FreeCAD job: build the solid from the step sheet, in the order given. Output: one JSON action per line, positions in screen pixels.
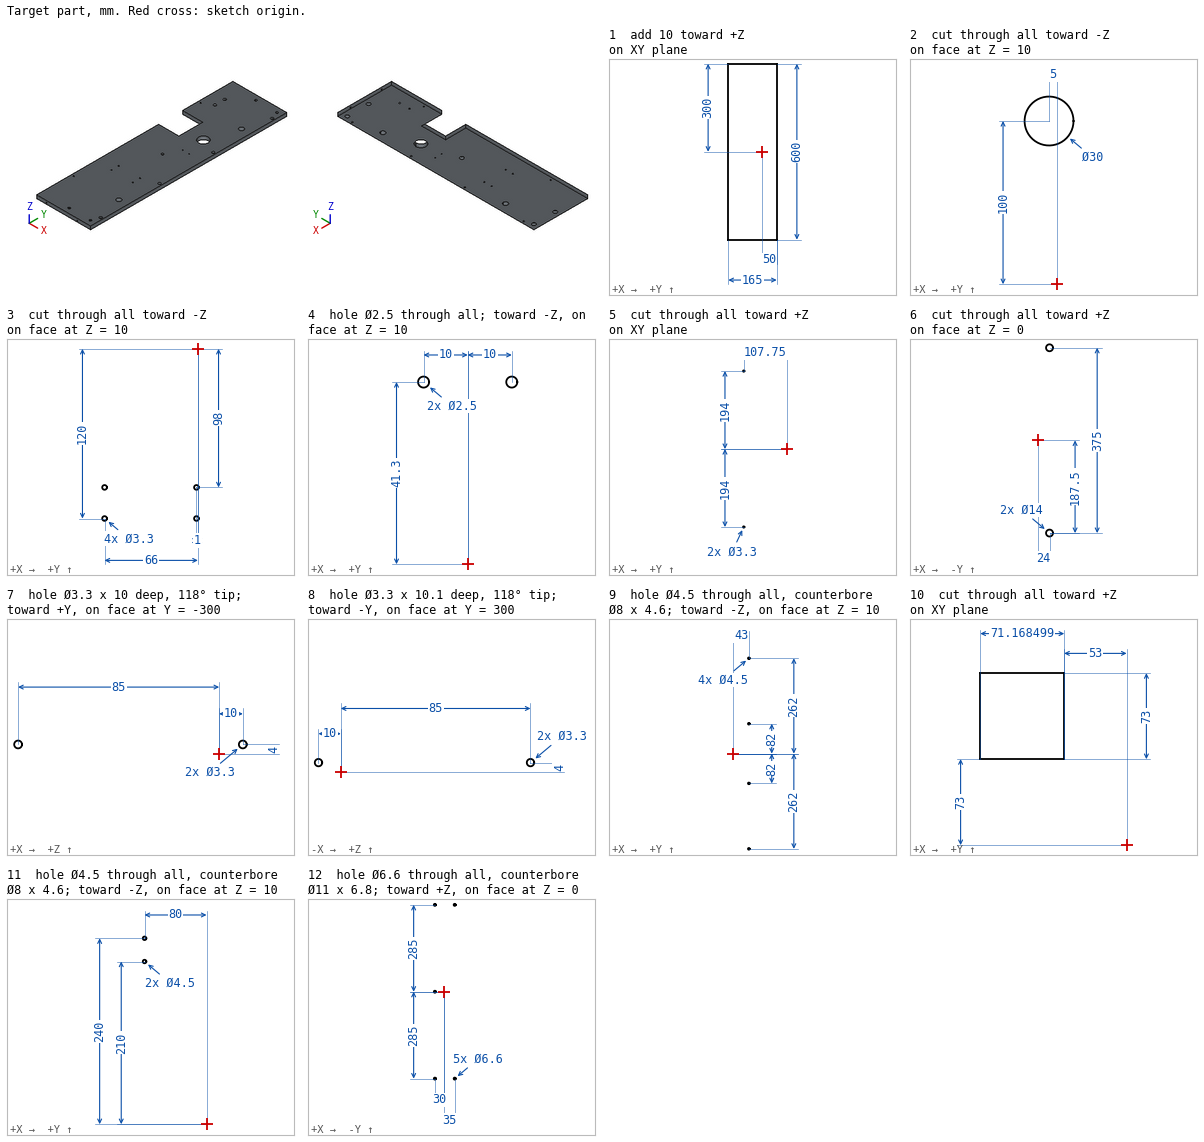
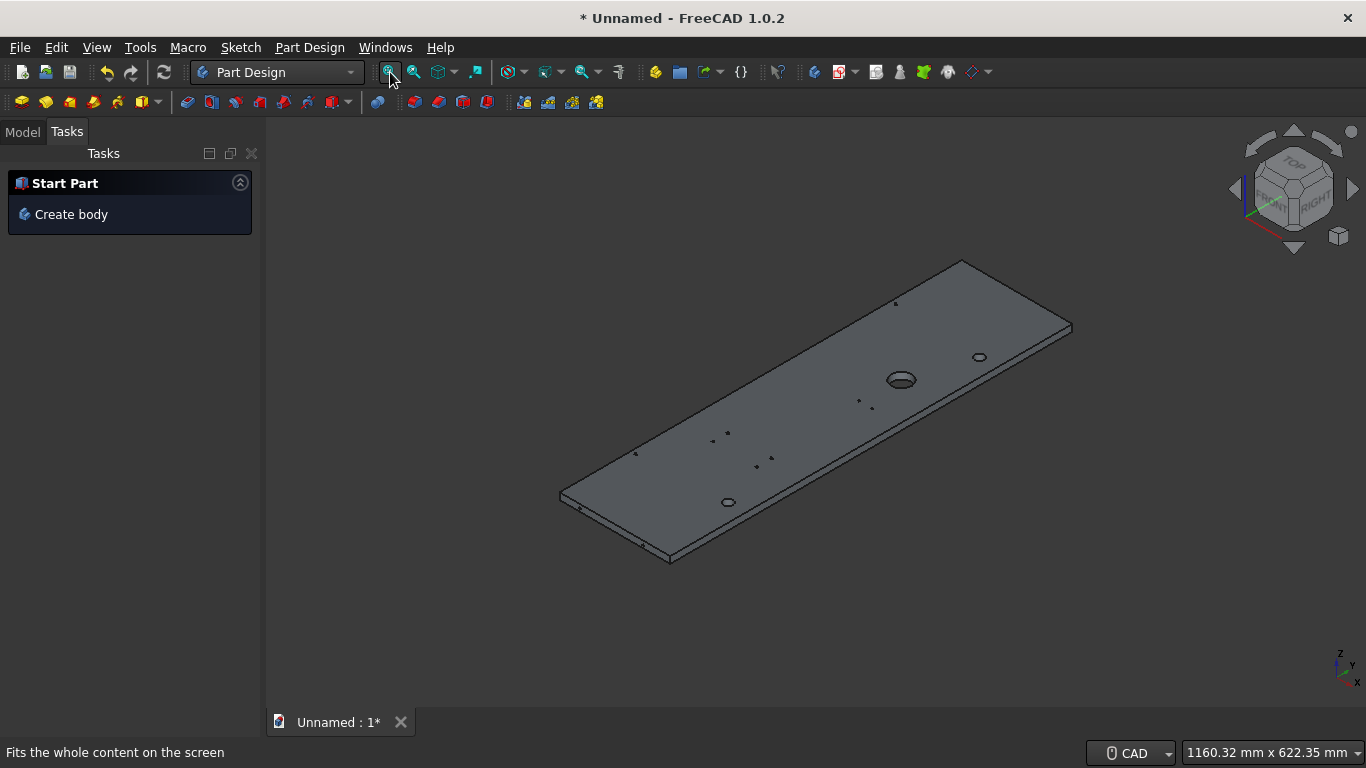
{"action": "left_click", "coordinate": [800, 398]}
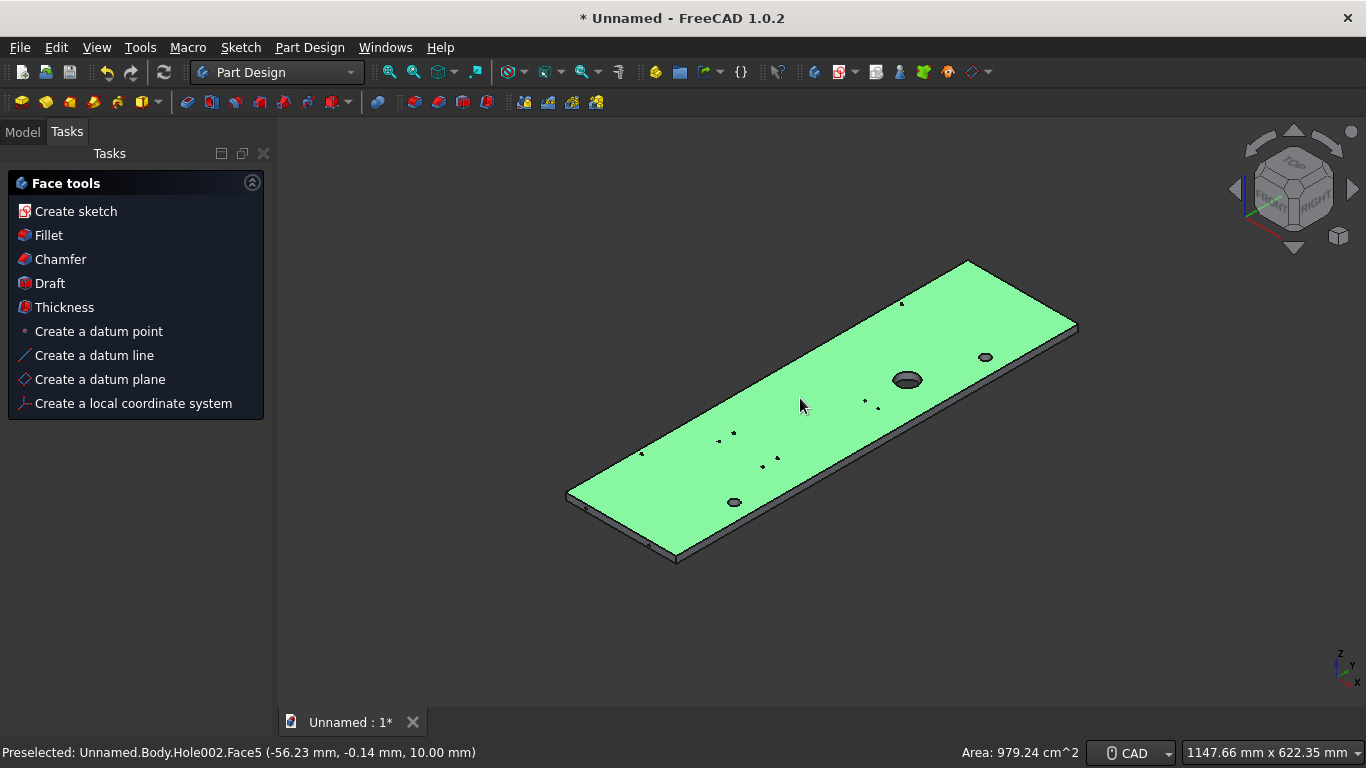
{"action": "left_click", "coordinate": [840, 72]}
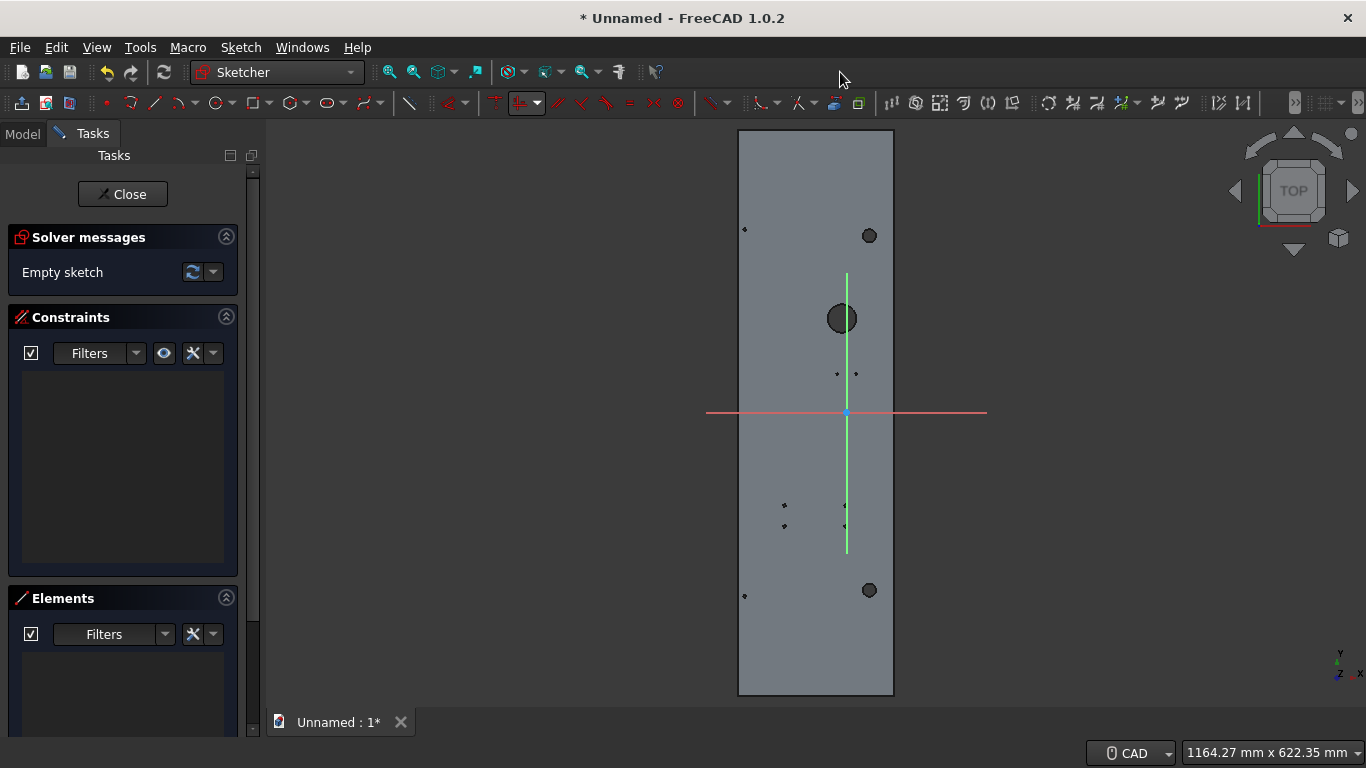
{"action": "scroll", "coordinate": [294, 413], "scroll_direction": "down", "scroll_amount": 1}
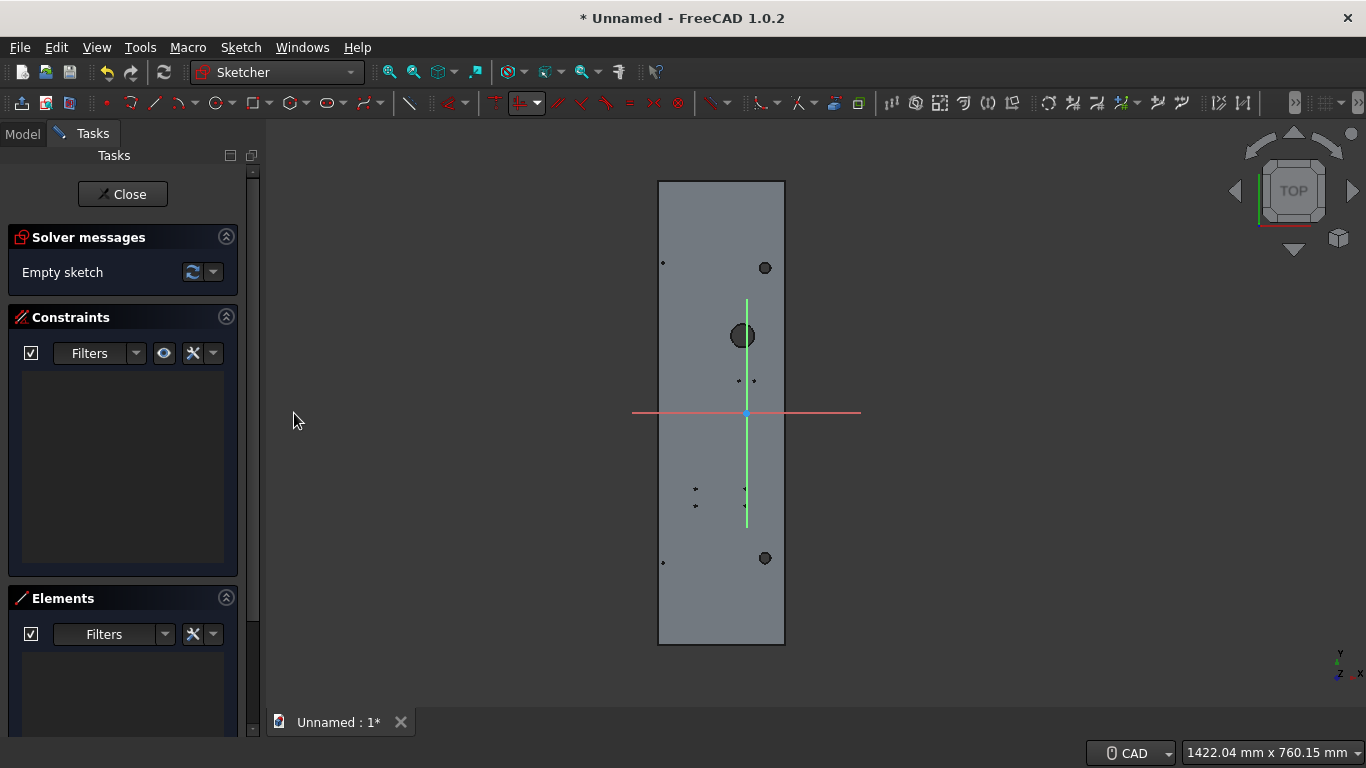
{"action": "left_click", "coordinate": [216, 104]}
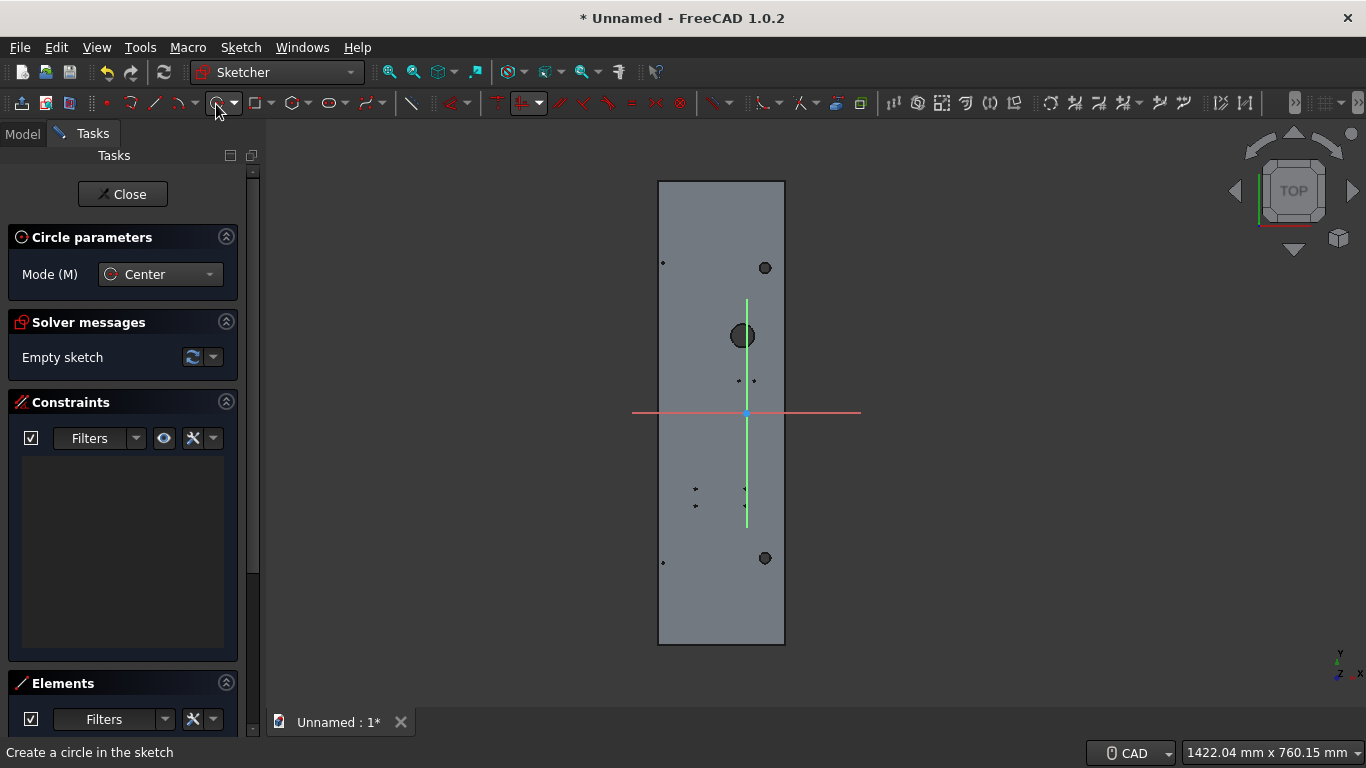
{"action": "scroll", "coordinate": [780, 210], "scroll_direction": "up", "scroll_amount": 13}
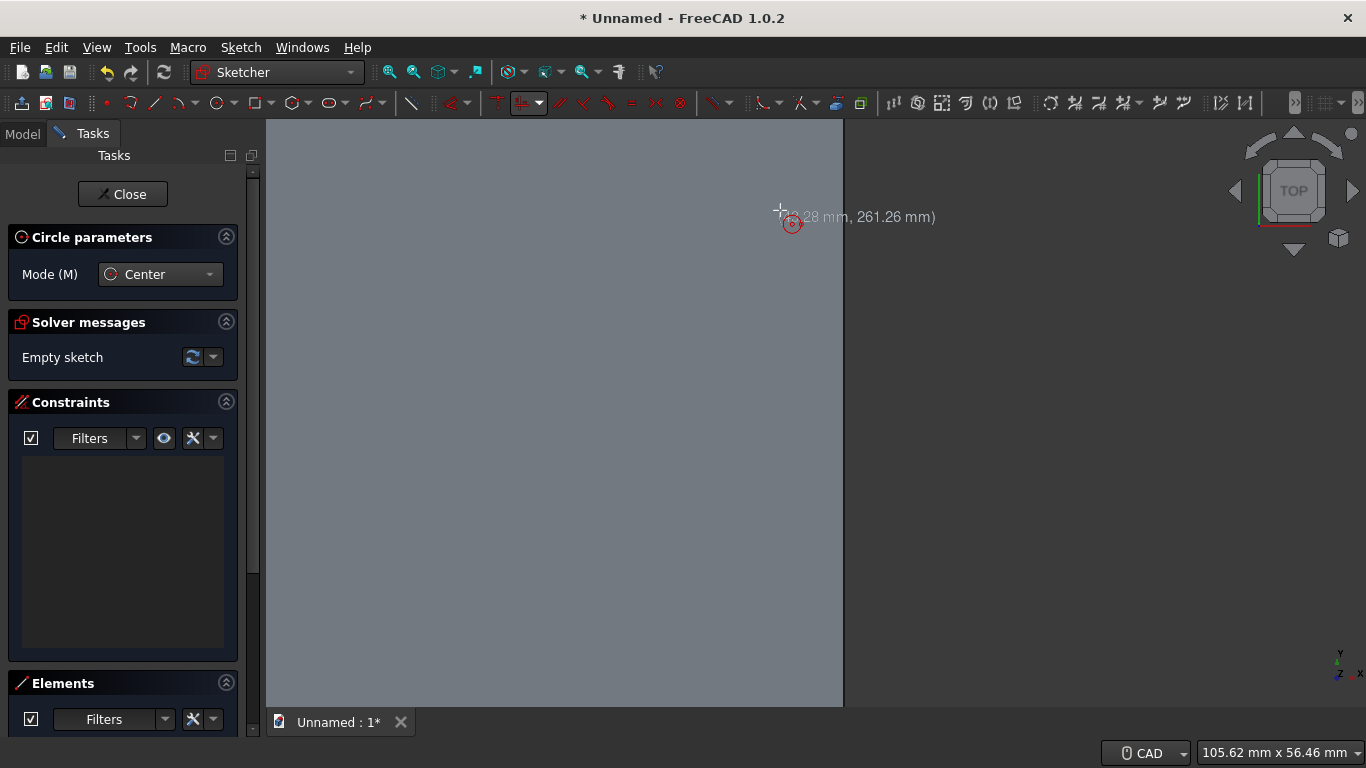
{"action": "scroll", "coordinate": [763, 210], "scroll_direction": "down", "scroll_amount": 13}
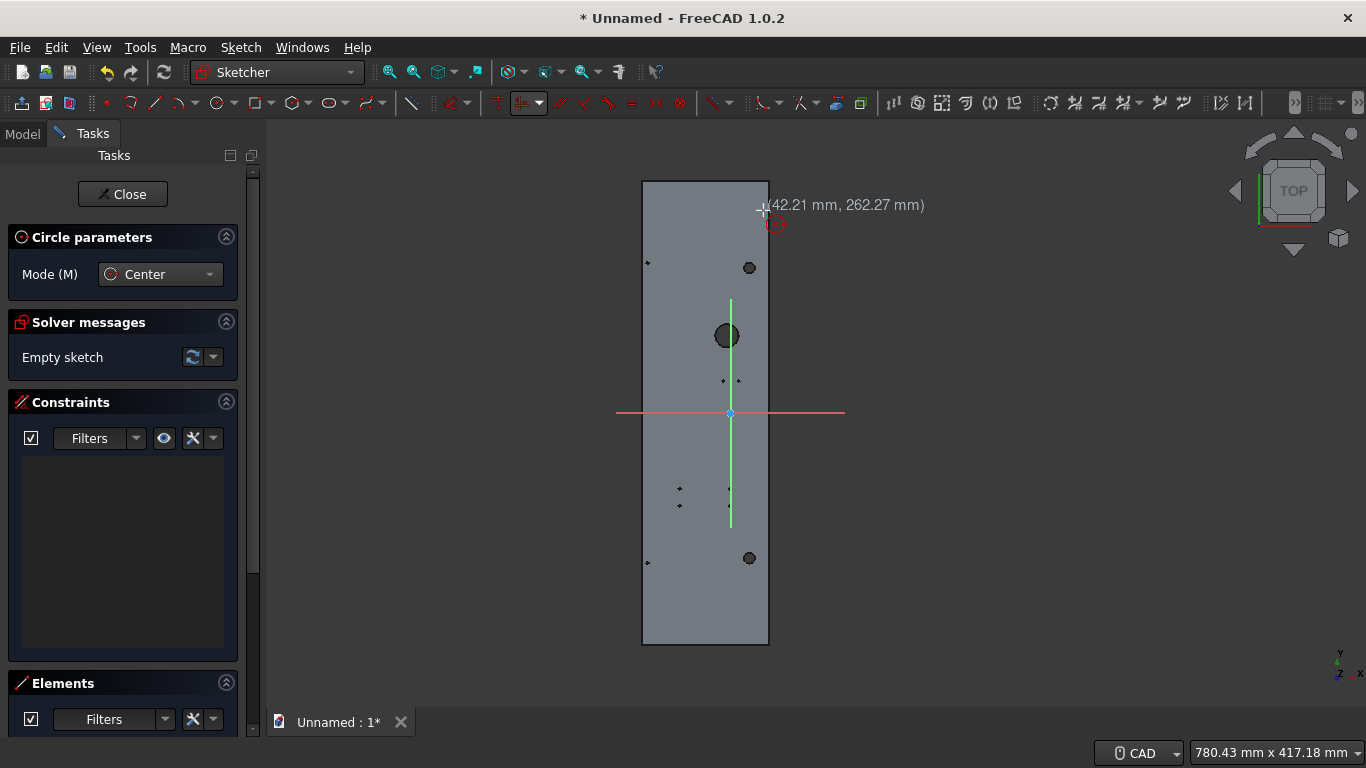
{"action": "left_click", "coordinate": [764, 210]}
{"action": "mouse_move", "coordinate": [765, 209]}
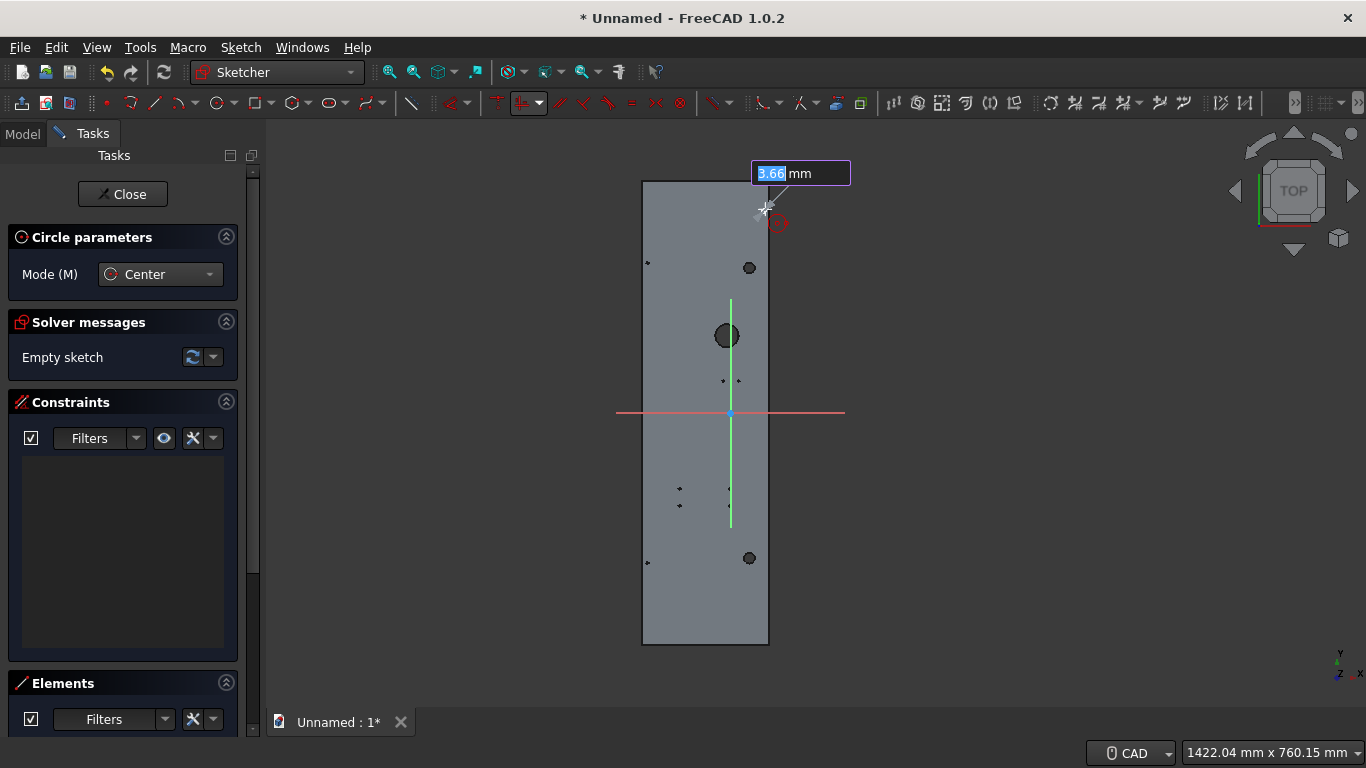
{"action": "type", "text": "4.5"}
{"action": "key", "text": "Return"}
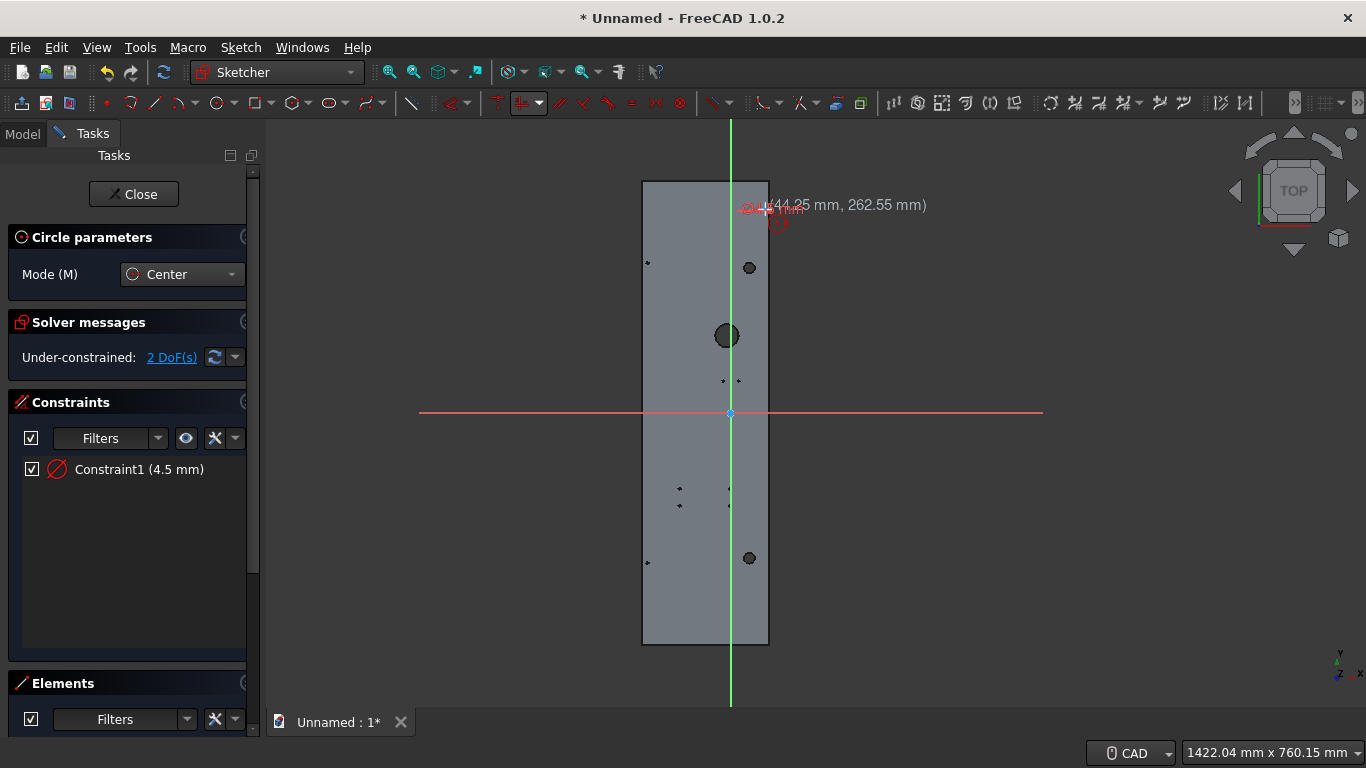
{"action": "scroll", "coordinate": [764, 350], "scroll_direction": "up", "scroll_amount": 13}